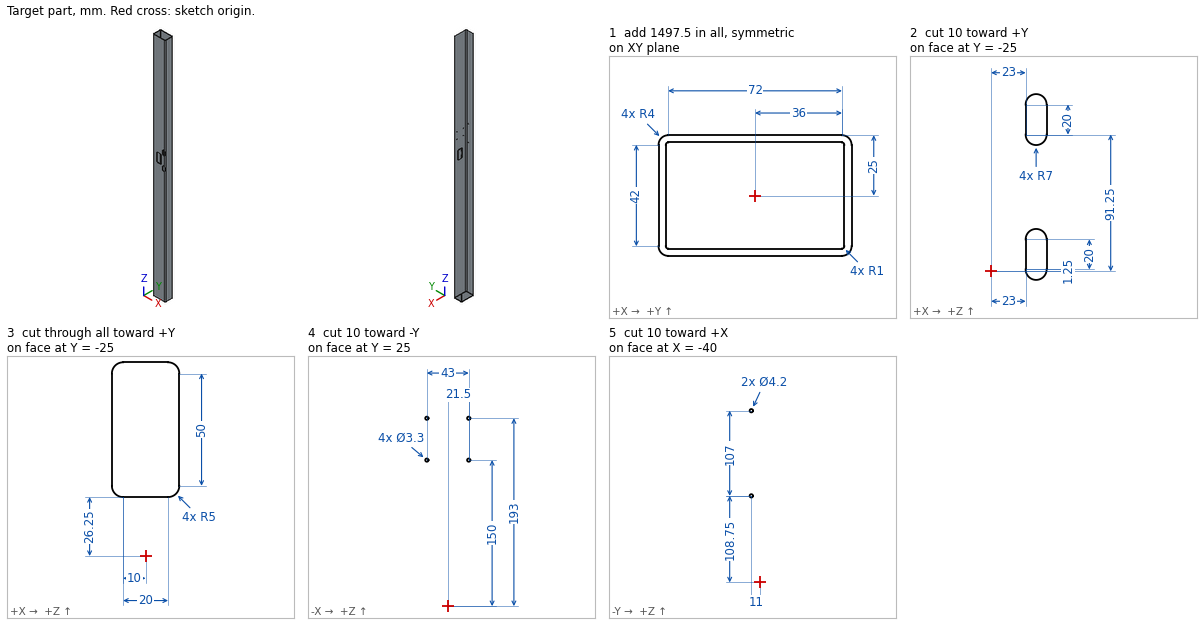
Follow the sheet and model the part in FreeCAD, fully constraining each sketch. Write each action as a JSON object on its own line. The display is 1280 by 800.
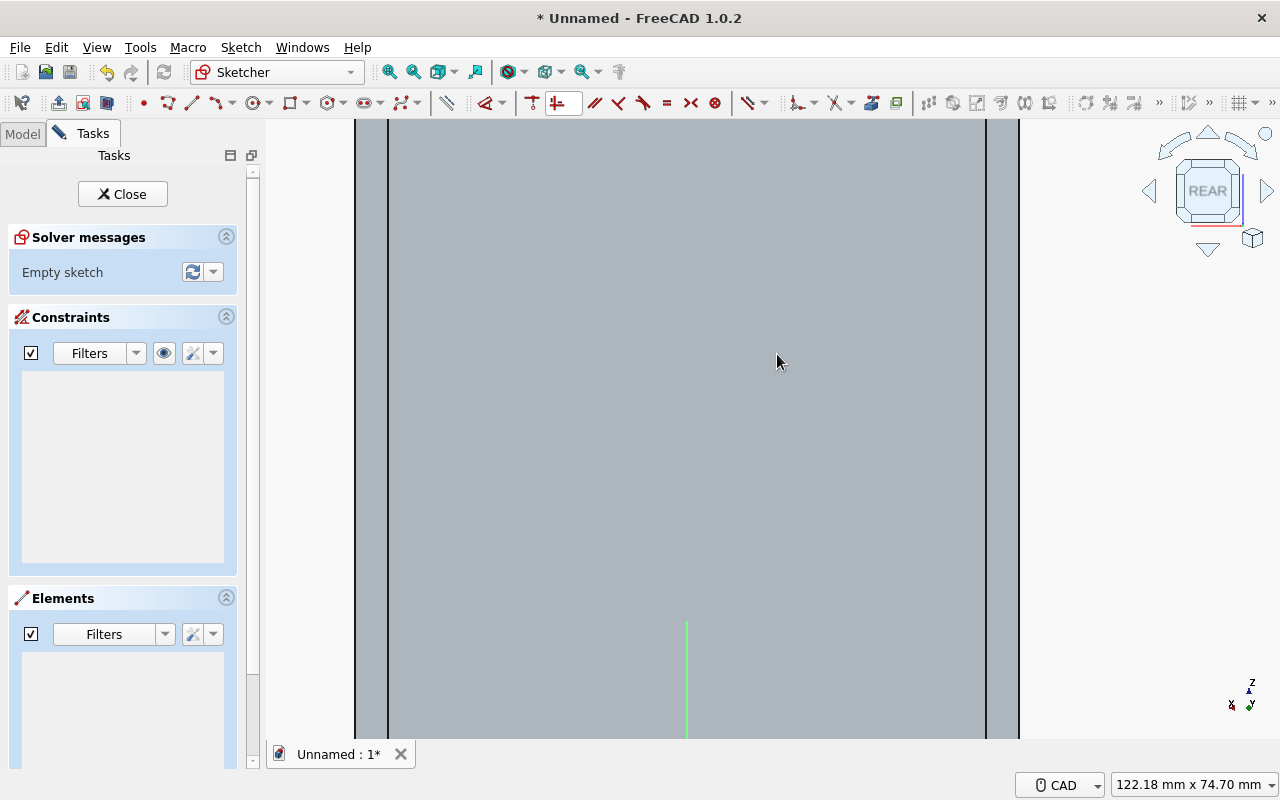
{"action": "left_click", "coordinate": [254, 104]}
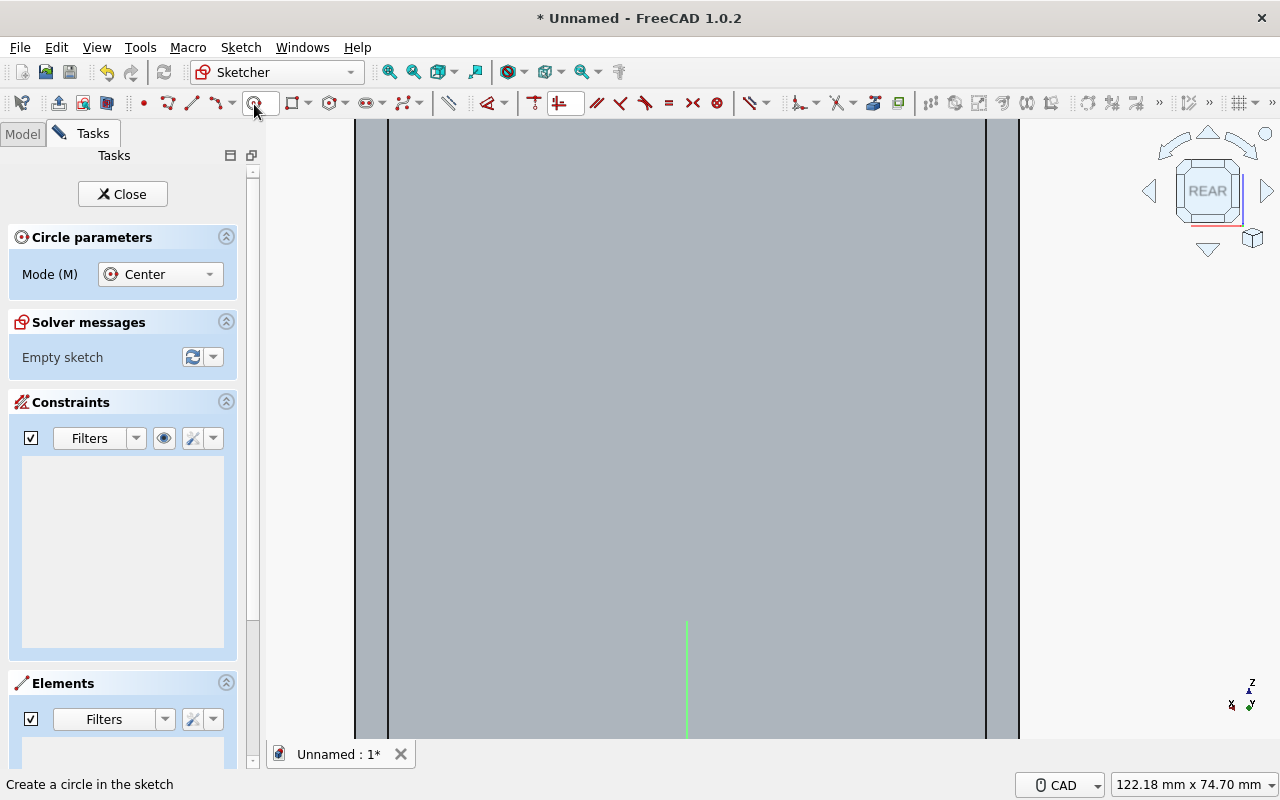
{"action": "scroll", "coordinate": [865, 608], "scroll_direction": "up", "scroll_amount": 3}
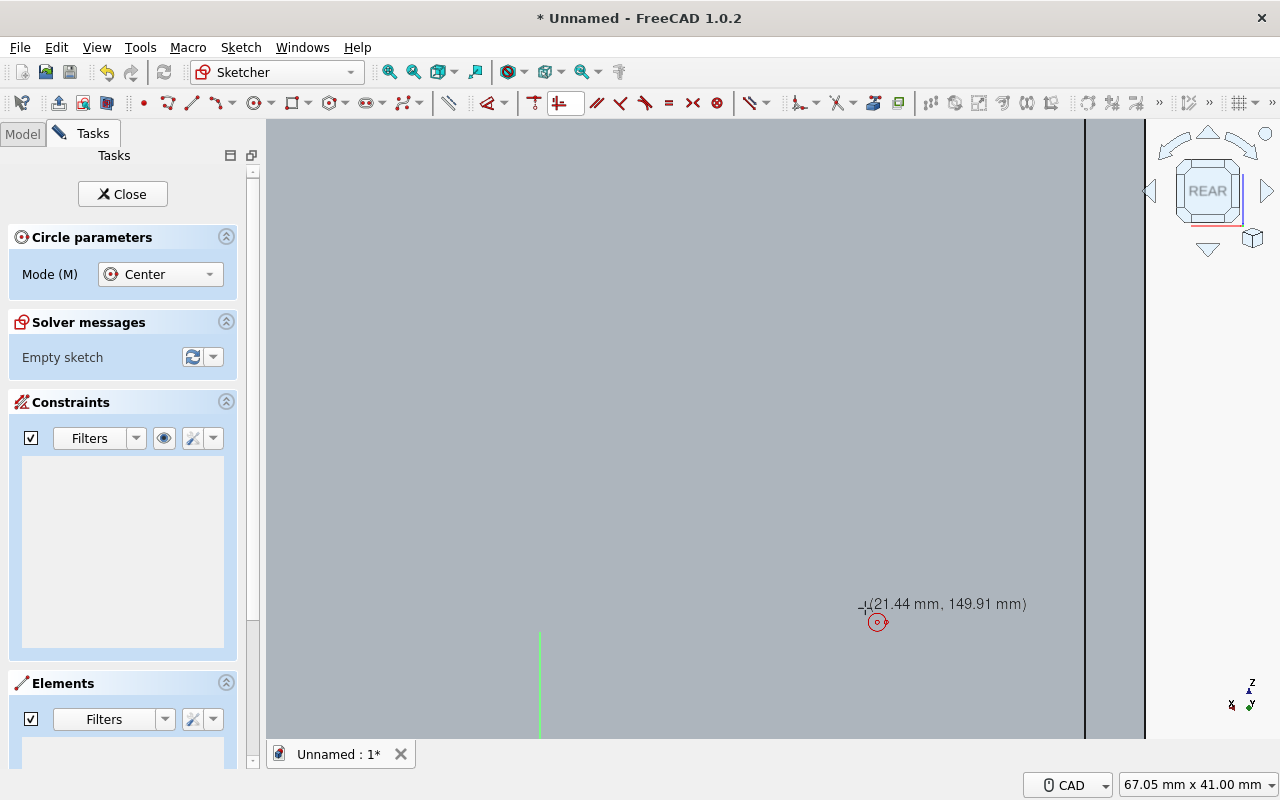
{"action": "left_click", "coordinate": [865, 608]}
{"action": "mouse_move", "coordinate": [883, 590]}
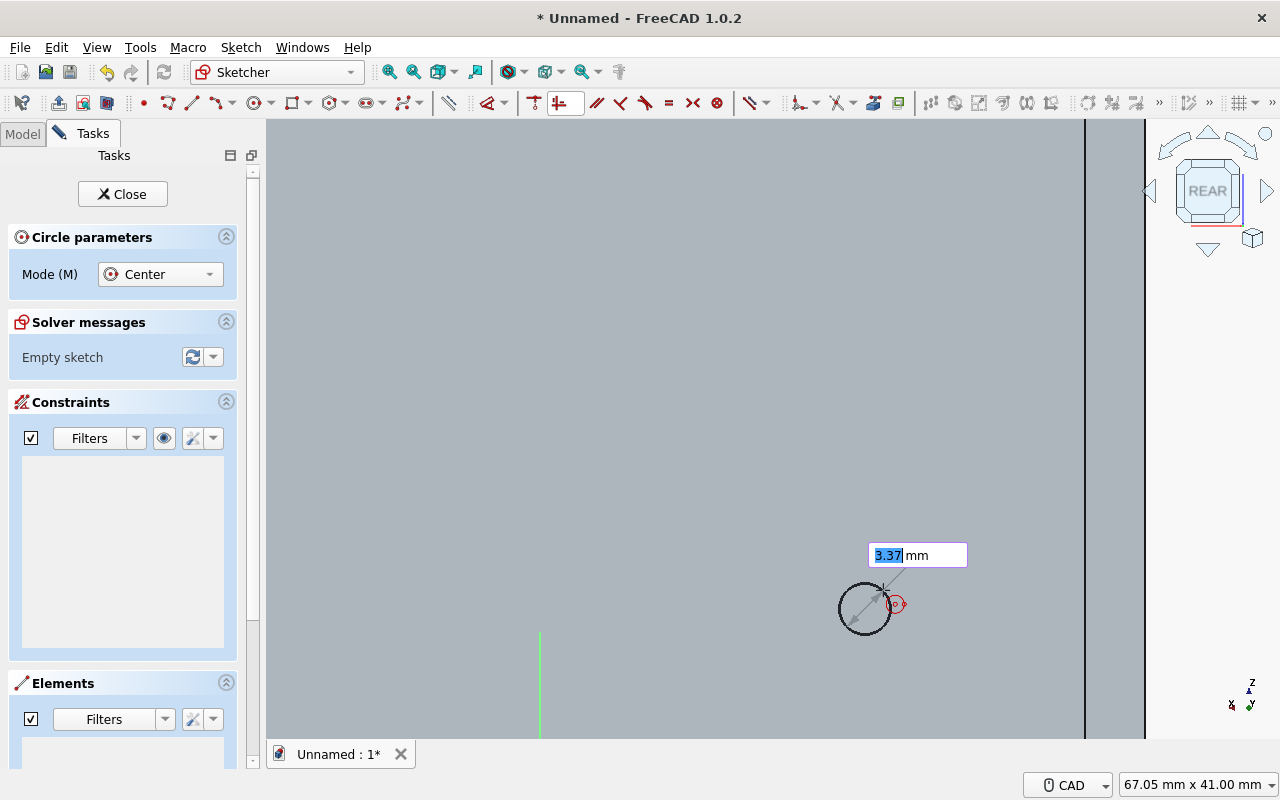
{"action": "type", "text": "3.3"}
{"action": "key", "text": "Return"}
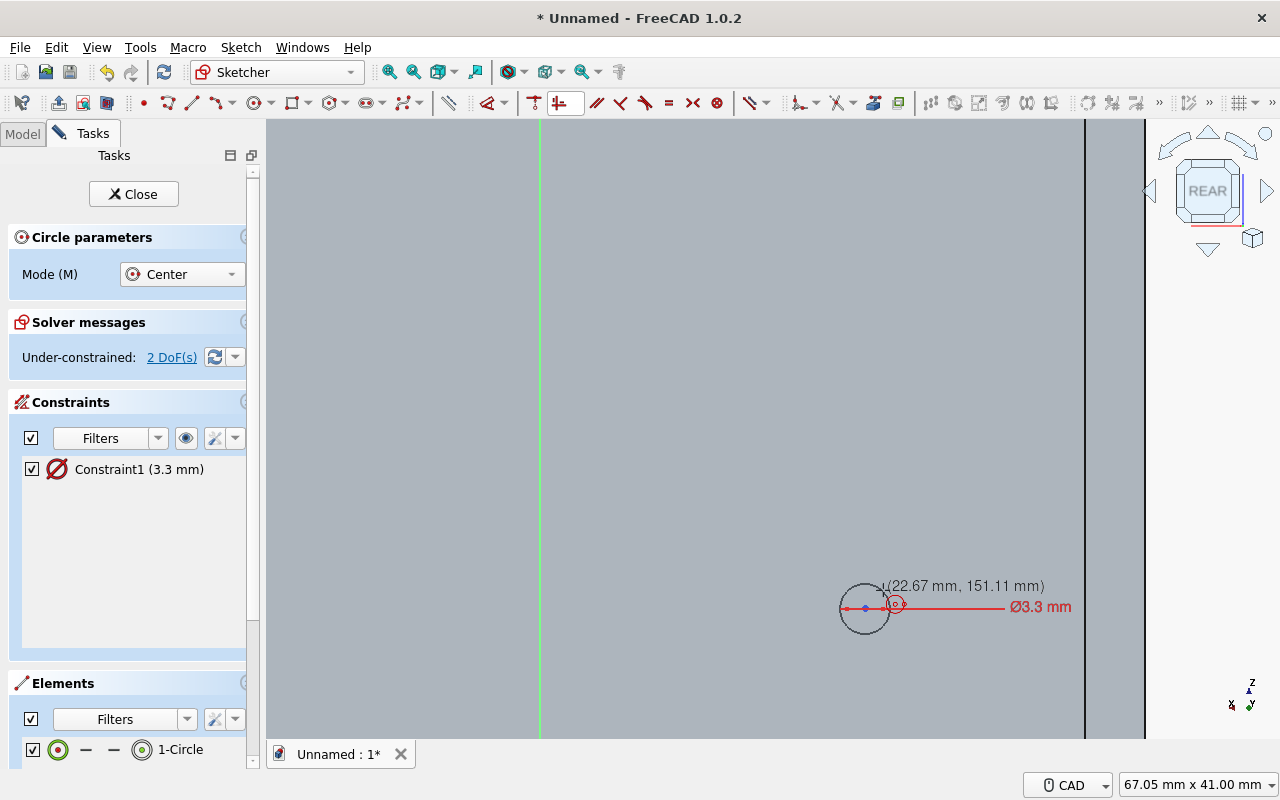
{"action": "scroll", "coordinate": [904, 607], "scroll_direction": "down", "scroll_amount": 3}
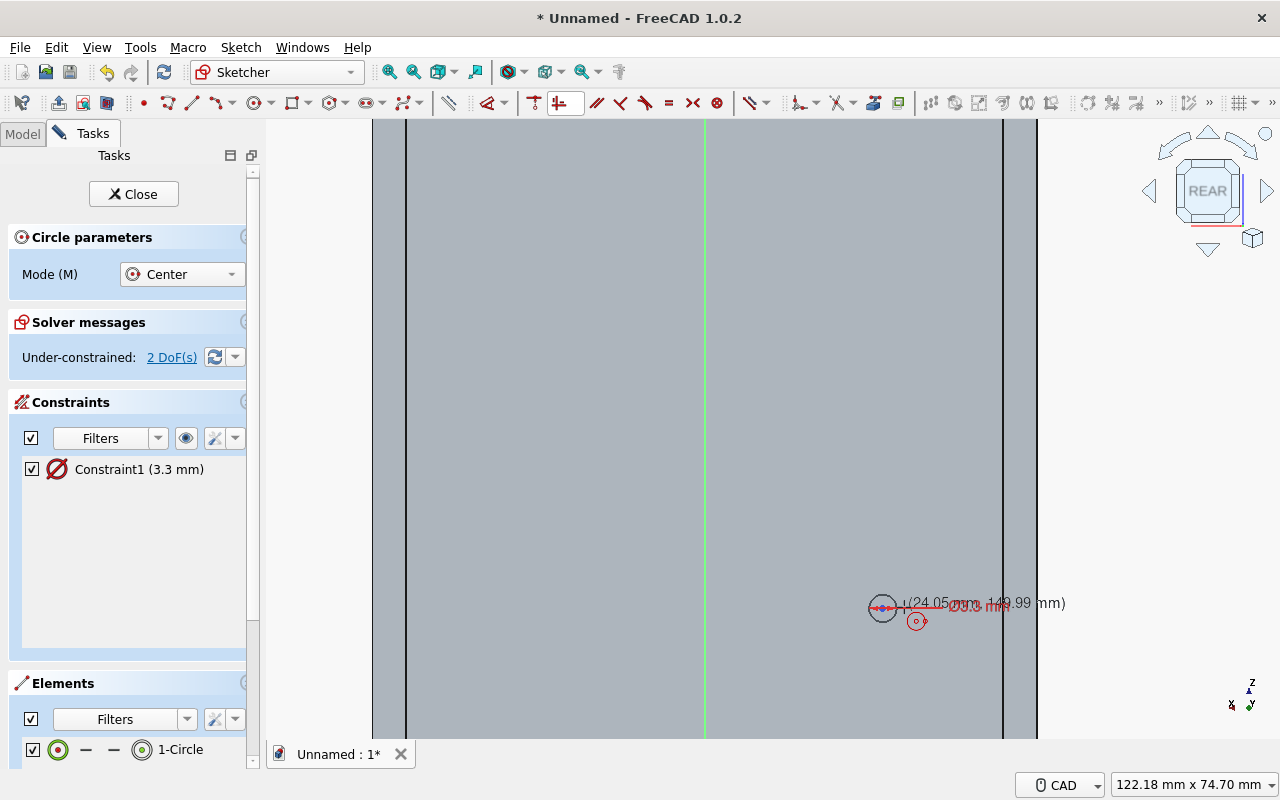
{"action": "scroll", "coordinate": [883, 251], "scroll_direction": "up", "scroll_amount": 3}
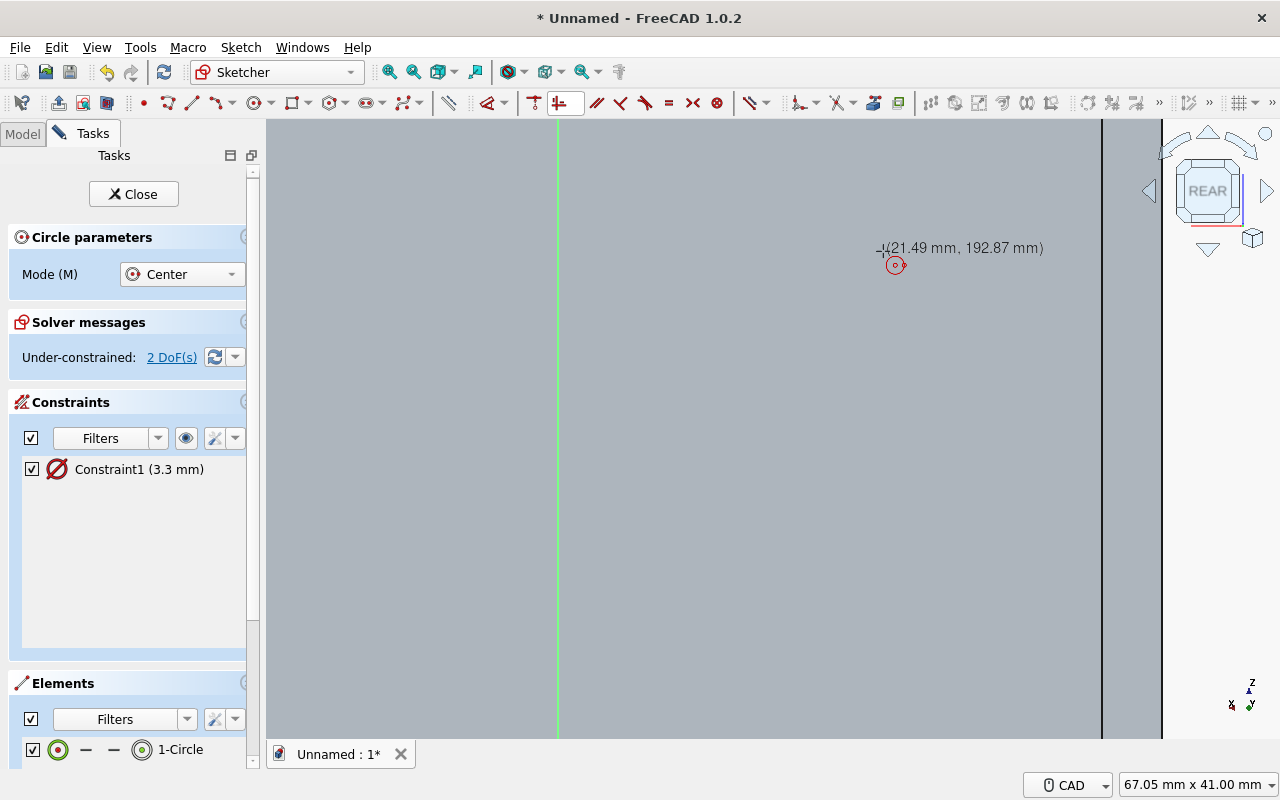
{"action": "left_click", "coordinate": [883, 251]}
{"action": "mouse_move", "coordinate": [900, 233]}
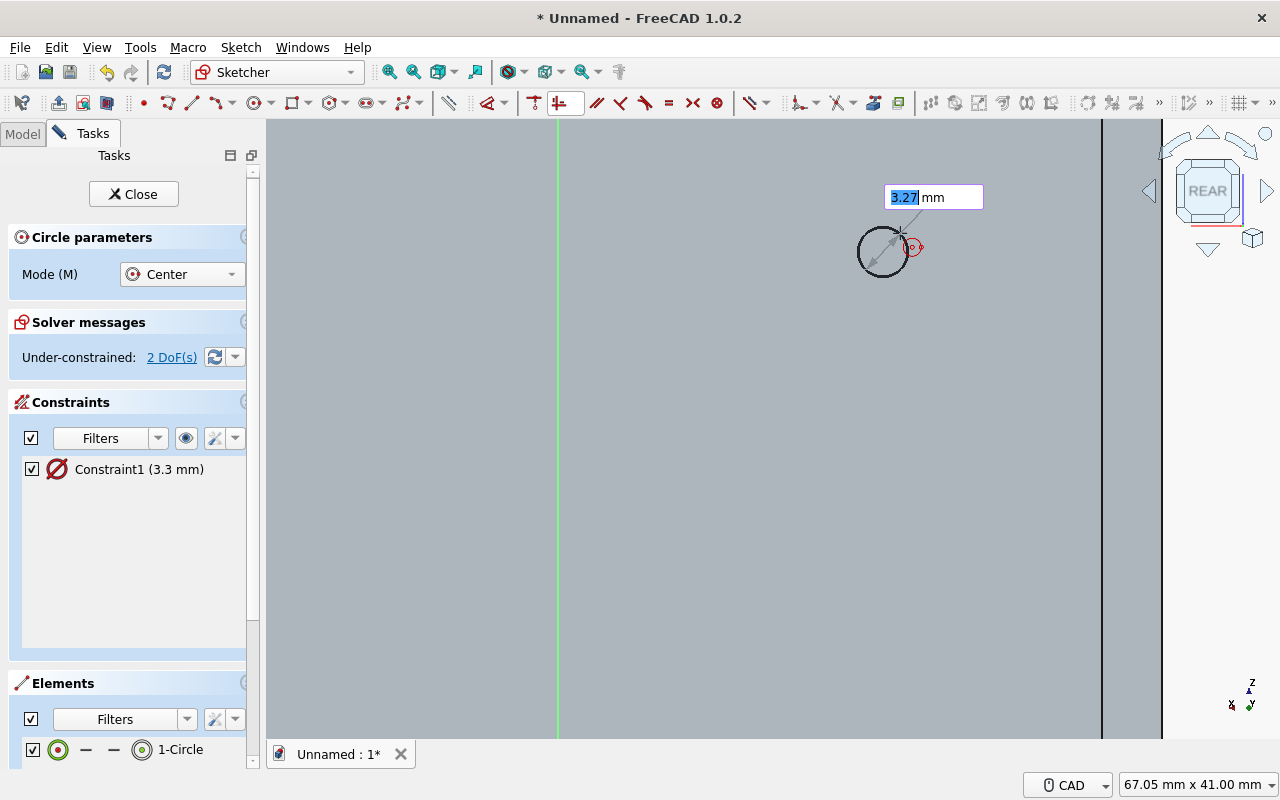
{"action": "type", "text": "3.3"}
{"action": "key", "text": "Return"}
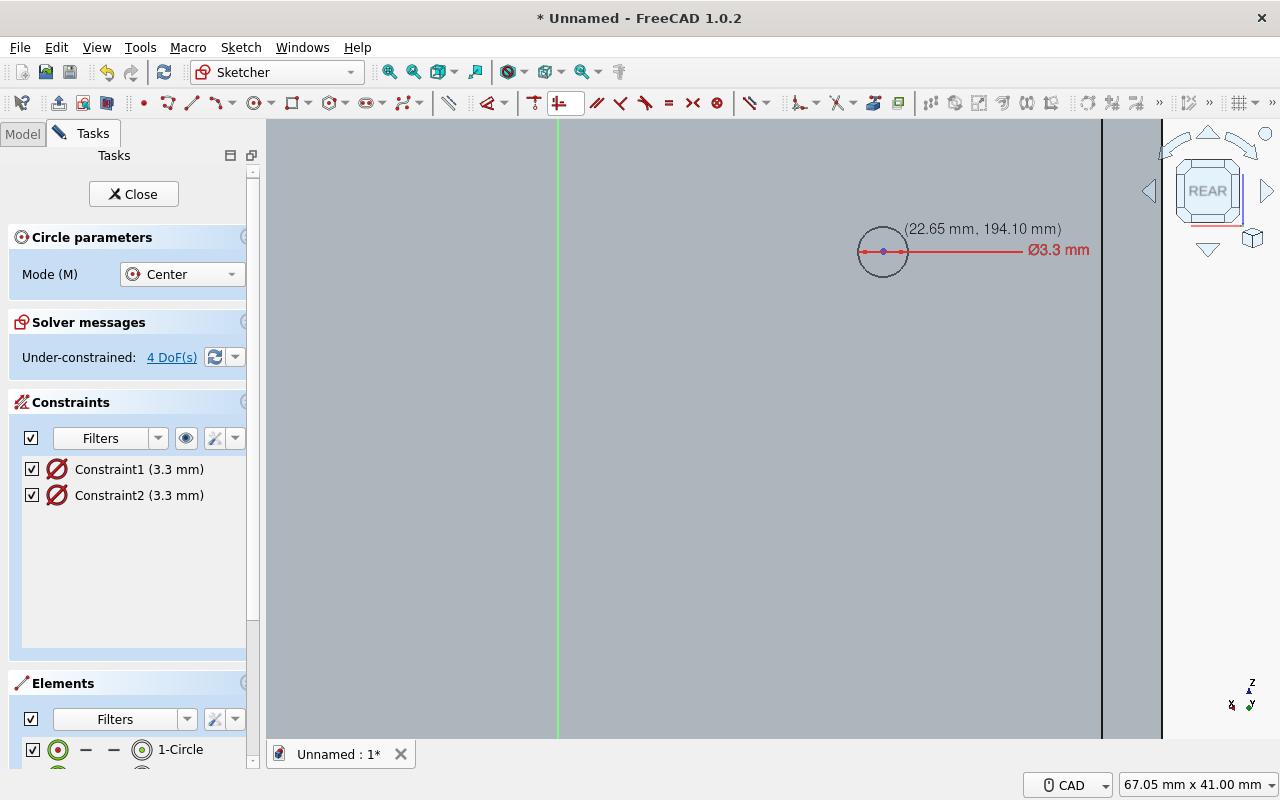
{"action": "scroll", "coordinate": [883, 250], "scroll_direction": "down", "scroll_amount": 3}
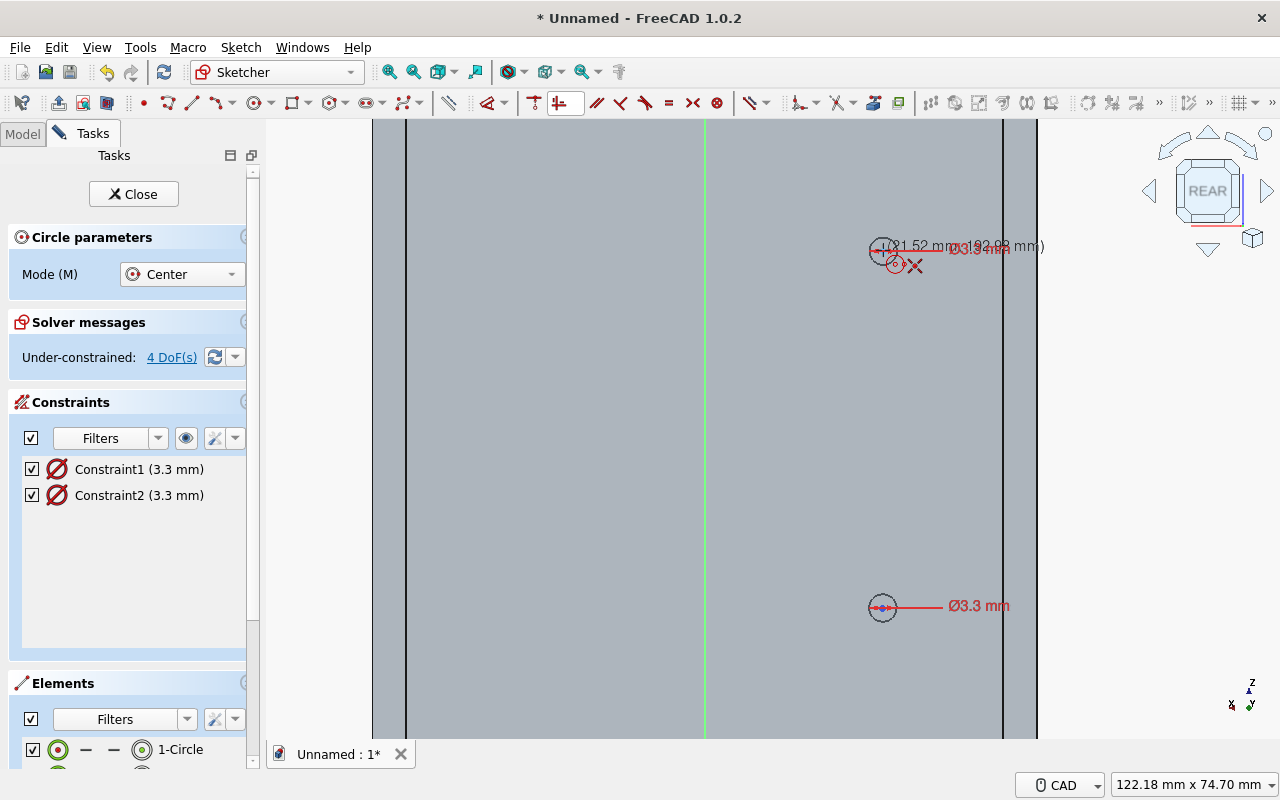
{"action": "scroll", "coordinate": [526, 607], "scroll_direction": "up", "scroll_amount": 3}